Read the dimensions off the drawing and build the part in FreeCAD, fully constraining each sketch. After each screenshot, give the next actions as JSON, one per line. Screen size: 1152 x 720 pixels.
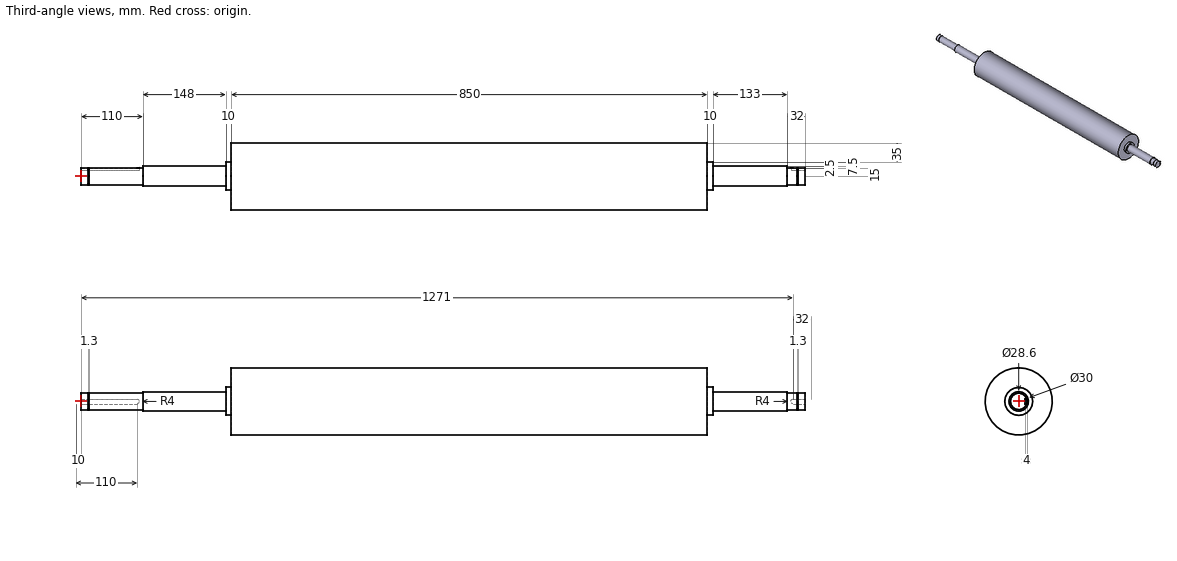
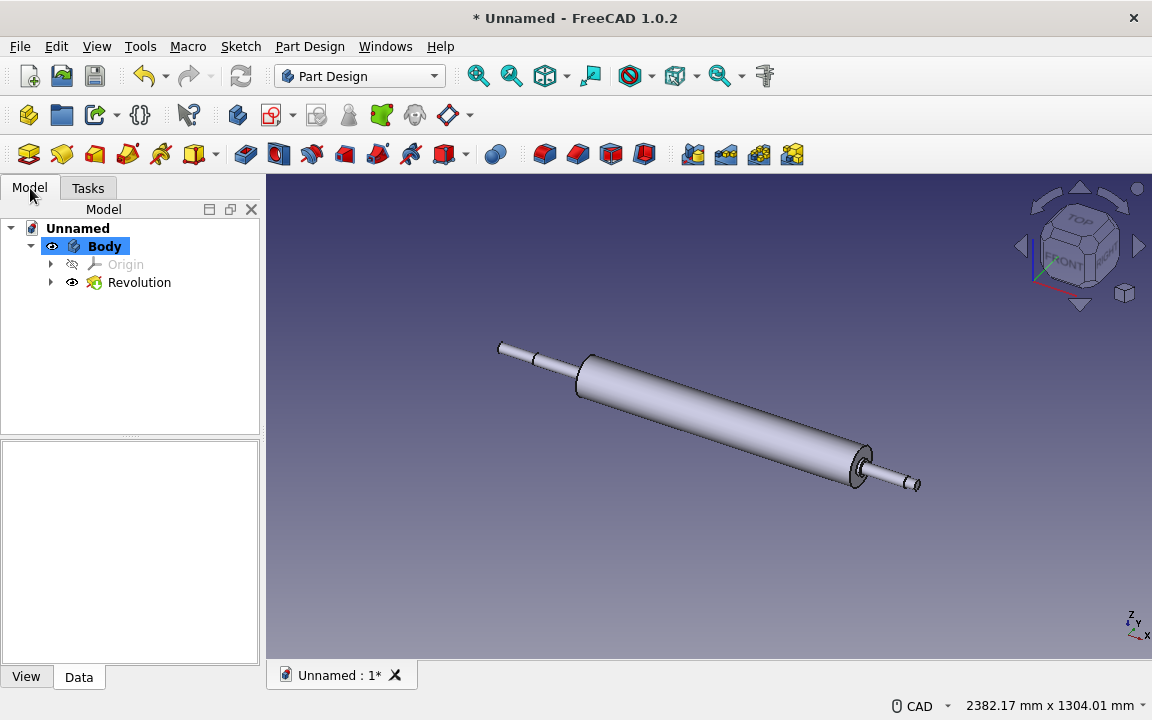
{"action": "left_click", "coordinate": [51, 264]}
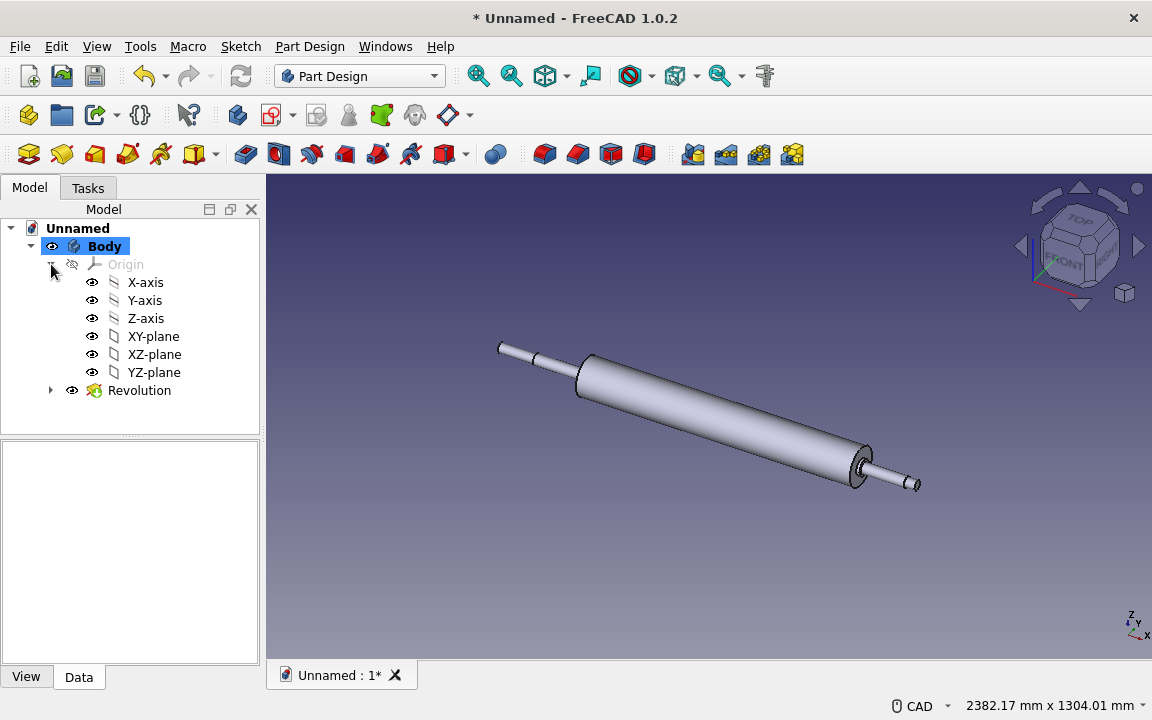
{"action": "left_click", "coordinate": [137, 354]}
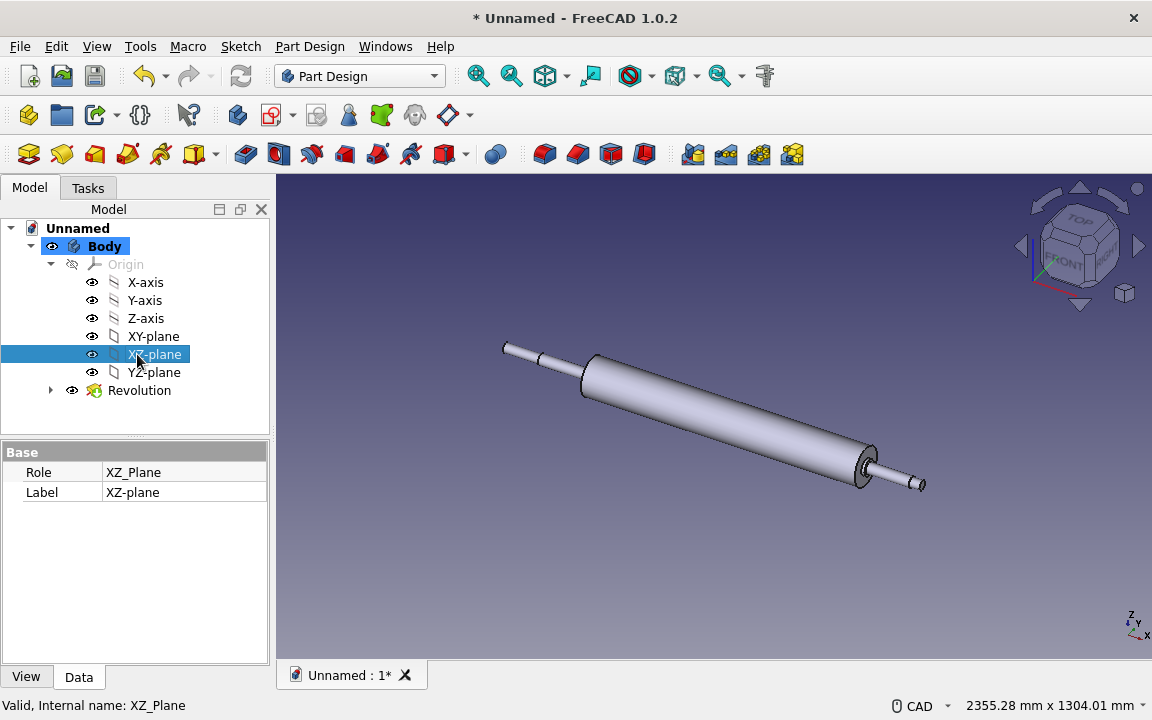
{"action": "left_click", "coordinate": [448, 116]}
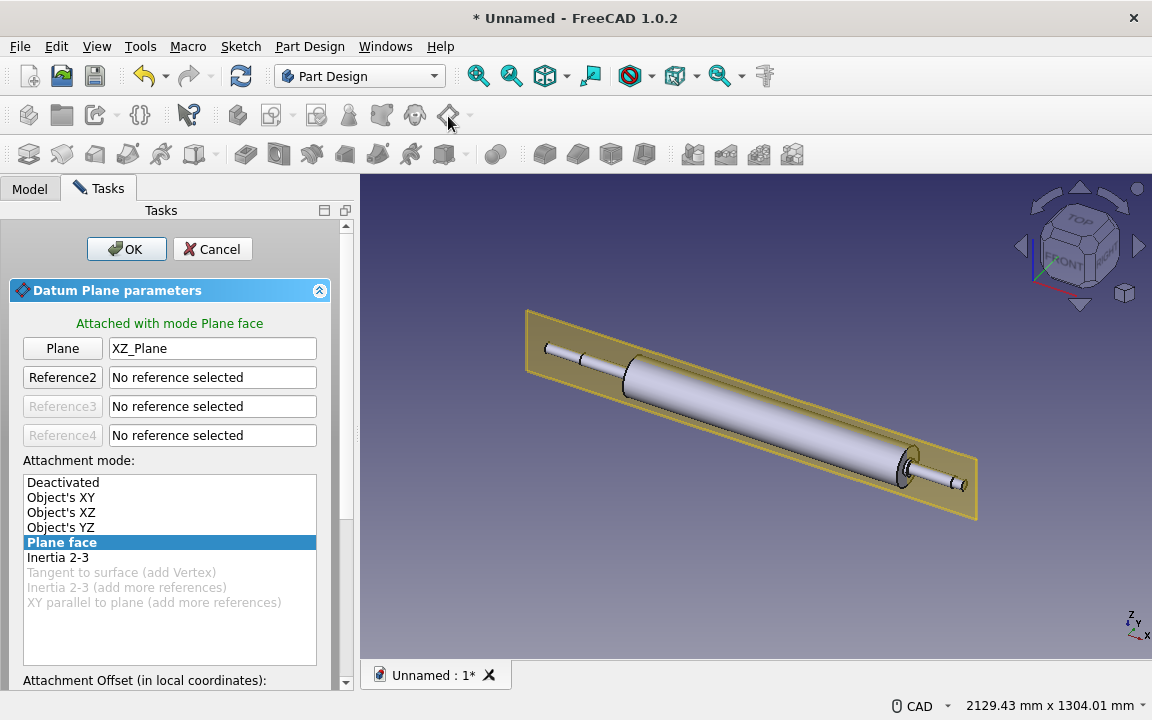
{"action": "scroll", "coordinate": [346, 455], "scroll_direction": "down", "scroll_amount": 3}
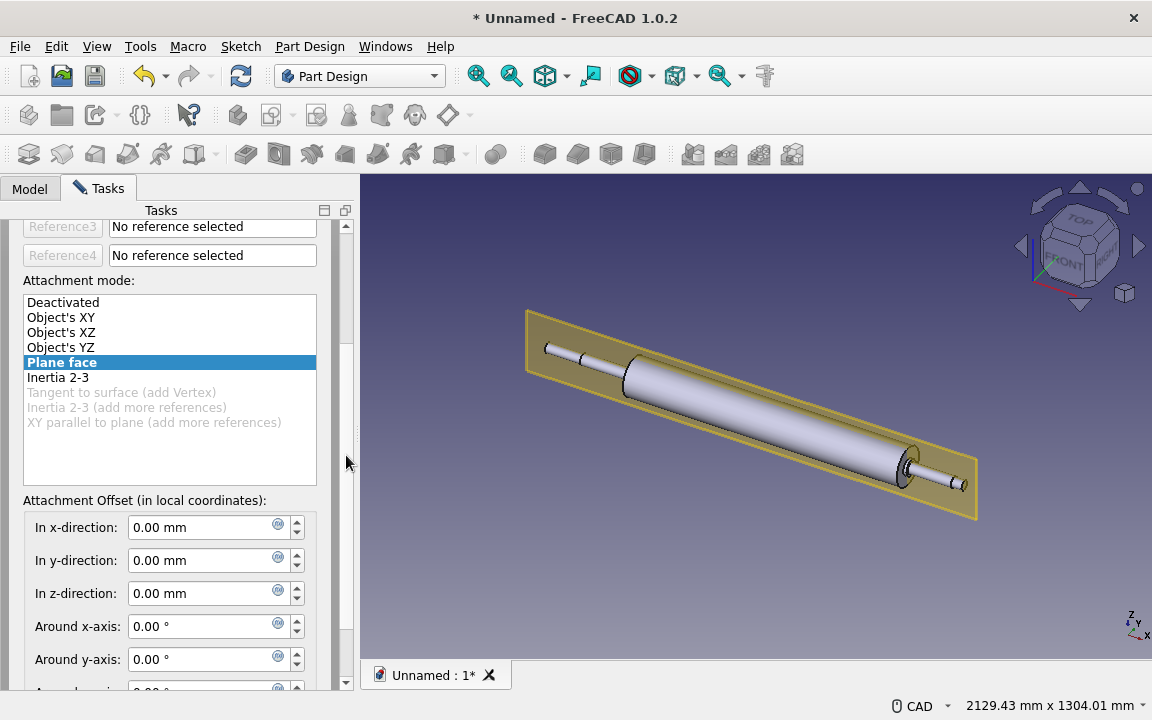
{"action": "triple_click", "coordinate": [210, 594]}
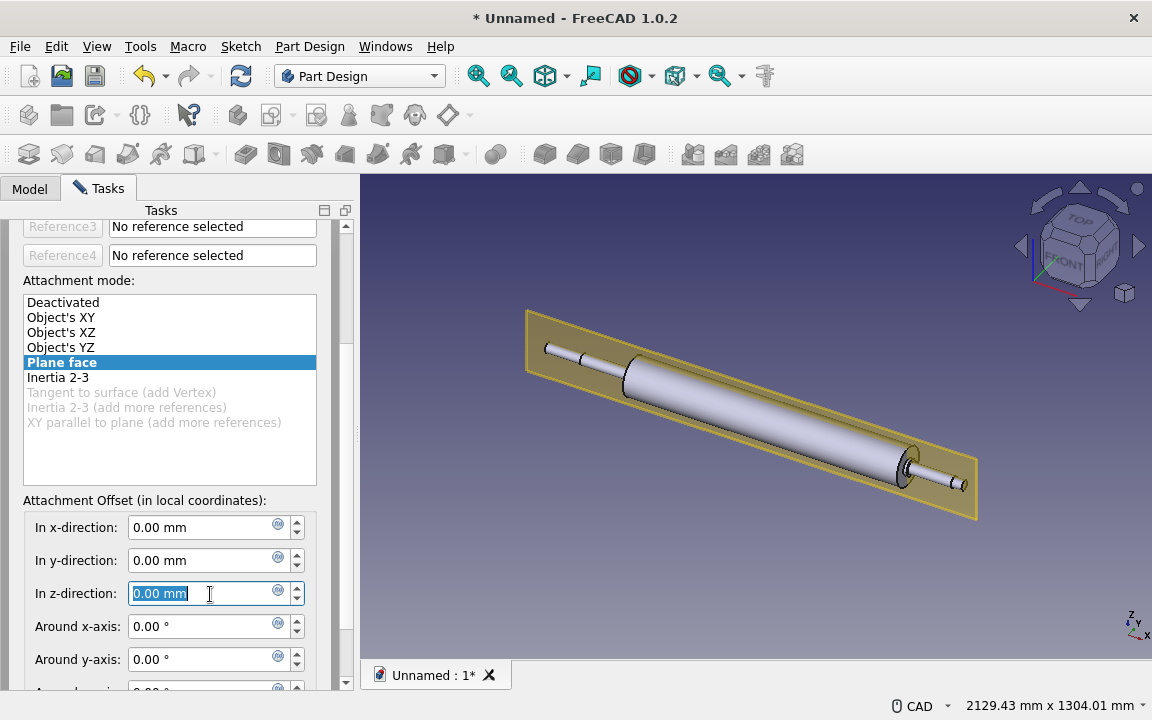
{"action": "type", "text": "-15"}
{"action": "key", "text": "Tab"}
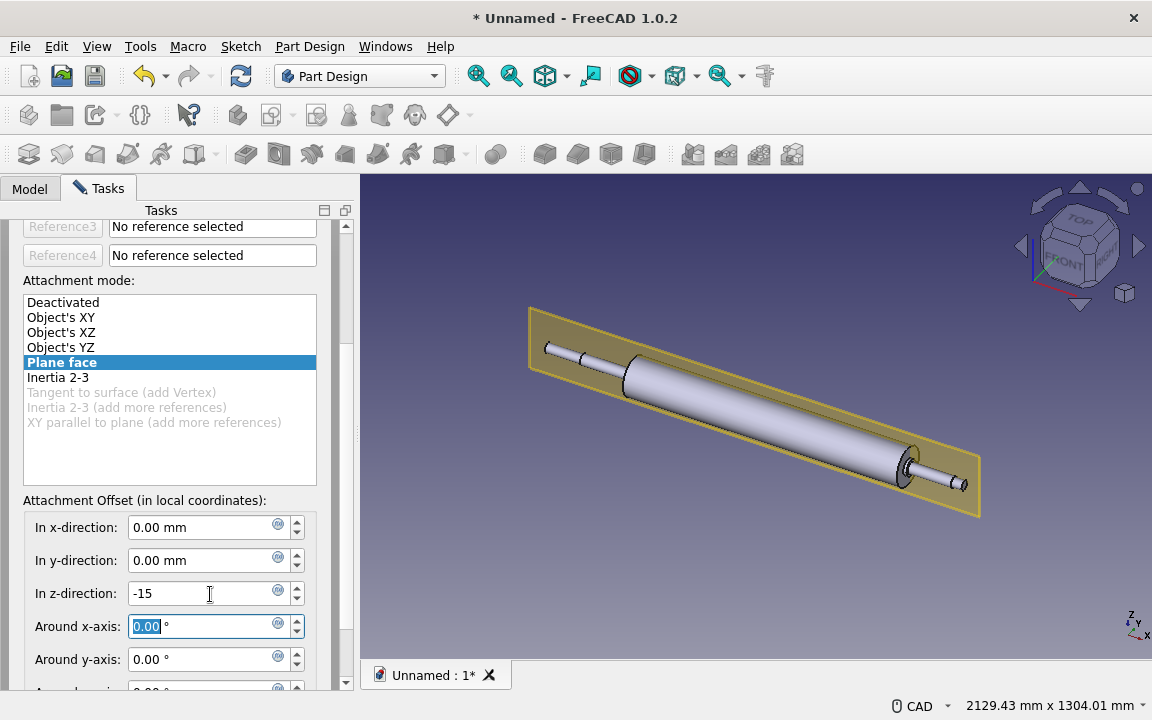
{"action": "scroll", "coordinate": [346, 455], "scroll_direction": "up", "scroll_amount": 4}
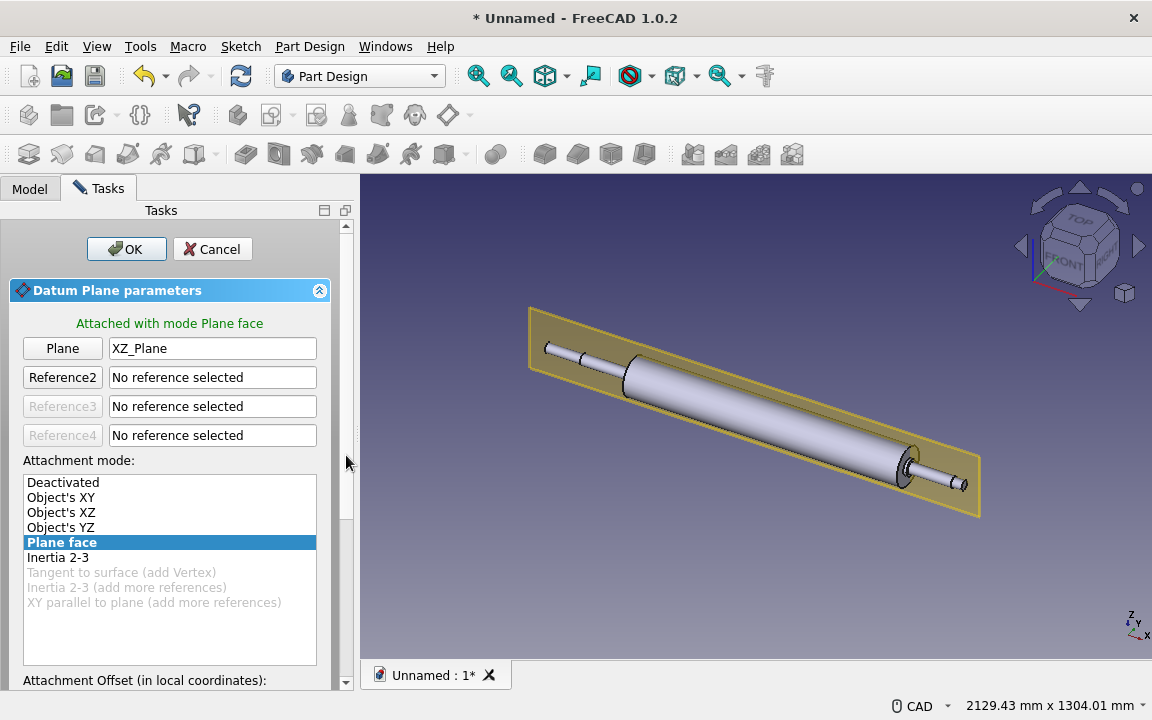
{"action": "left_click", "coordinate": [127, 249]}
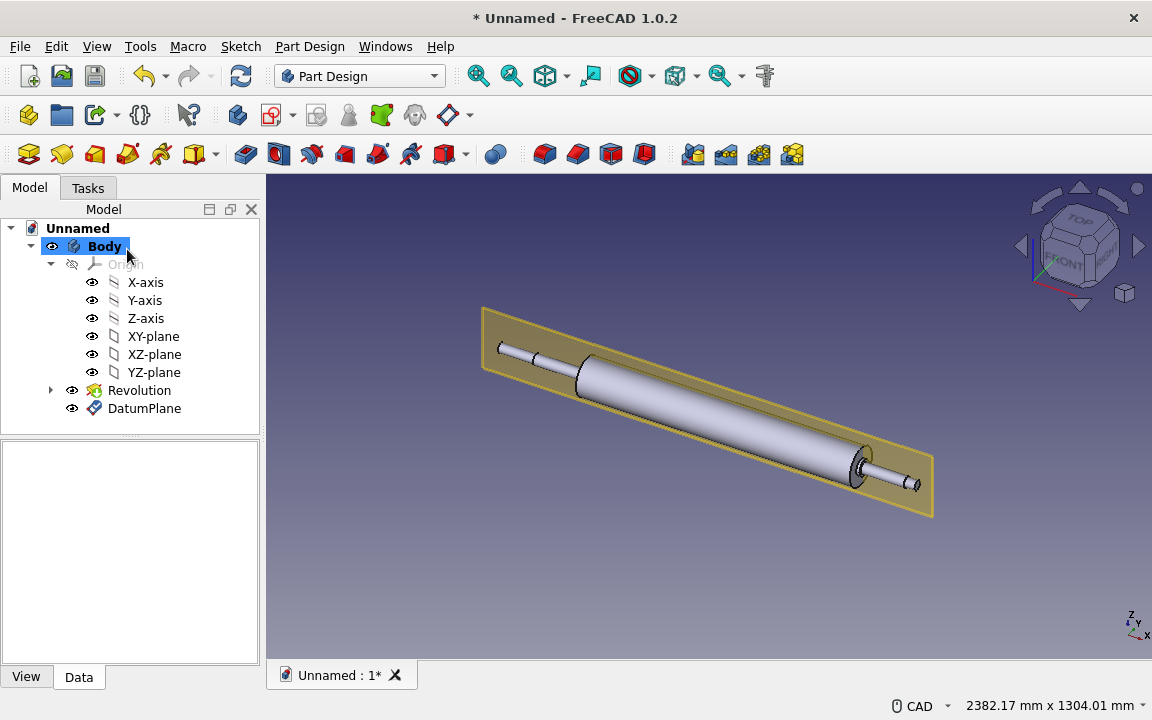
{"action": "left_click", "coordinate": [117, 408]}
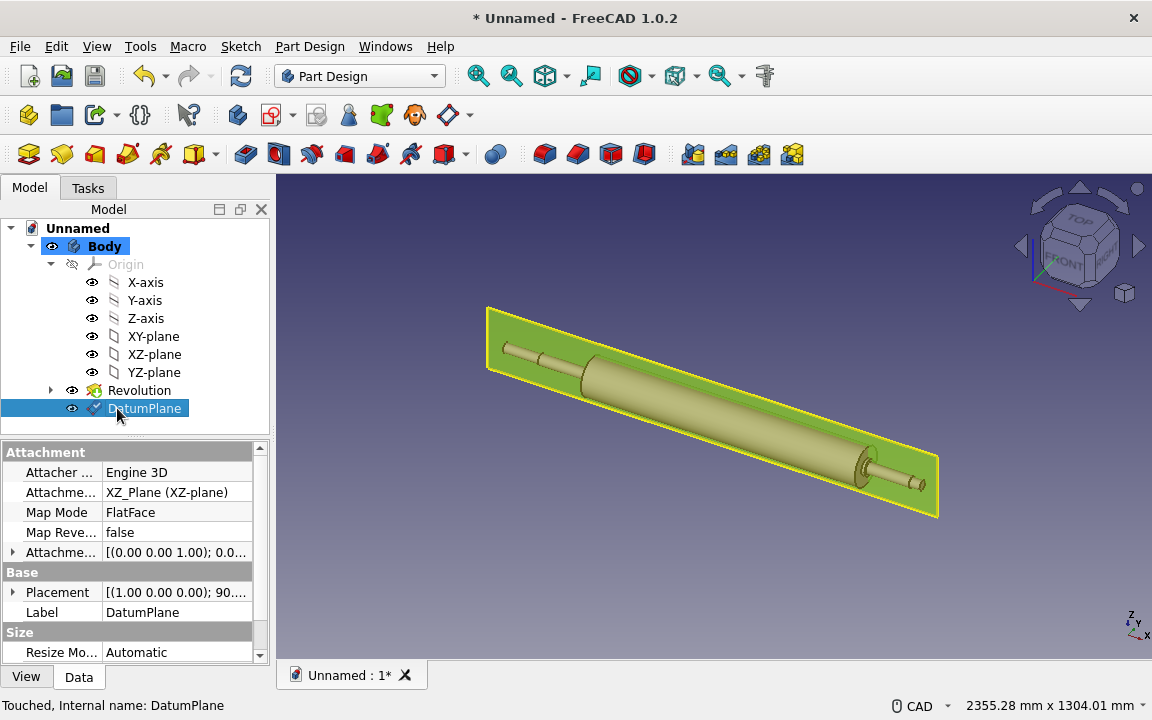
{"action": "left_click", "coordinate": [270, 116]}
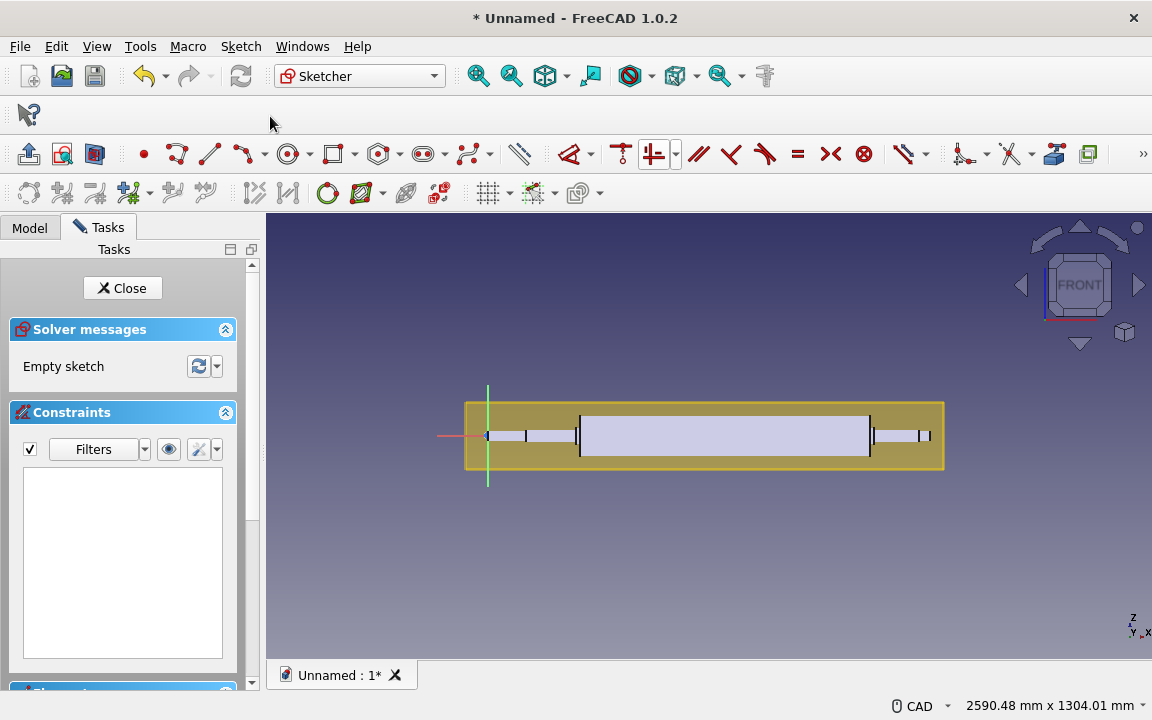
{"action": "key", "text": "q s"}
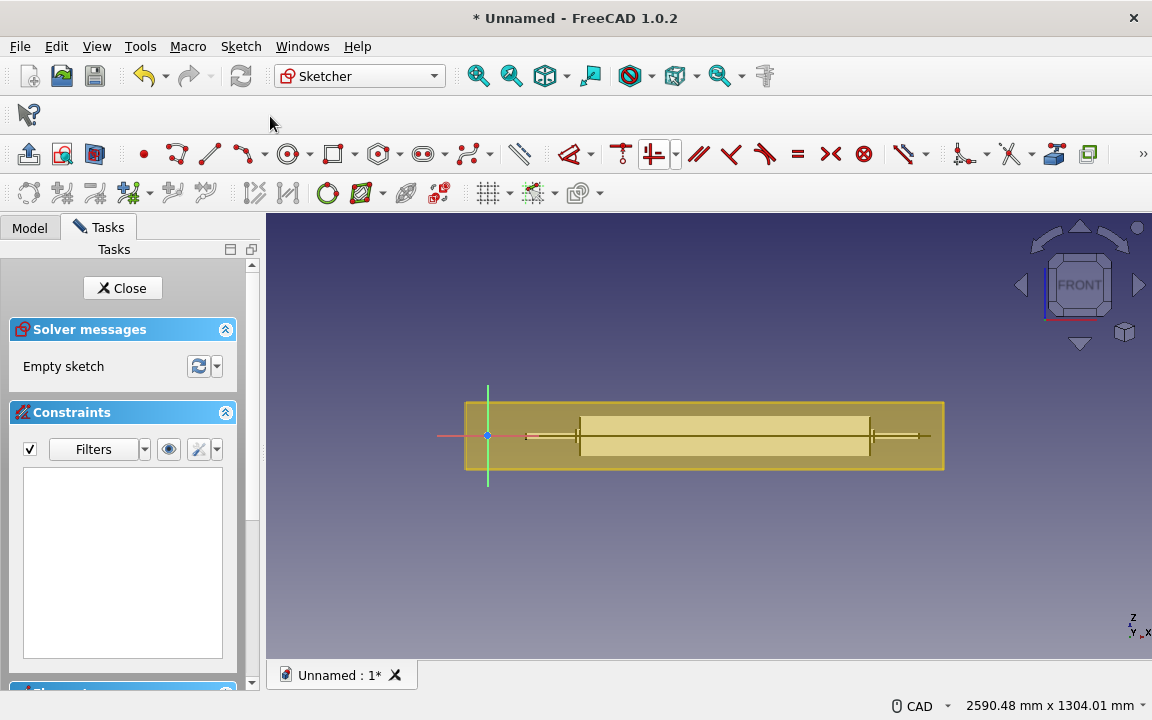
{"action": "scroll", "coordinate": [493, 436], "scroll_direction": "up", "scroll_amount": 13}